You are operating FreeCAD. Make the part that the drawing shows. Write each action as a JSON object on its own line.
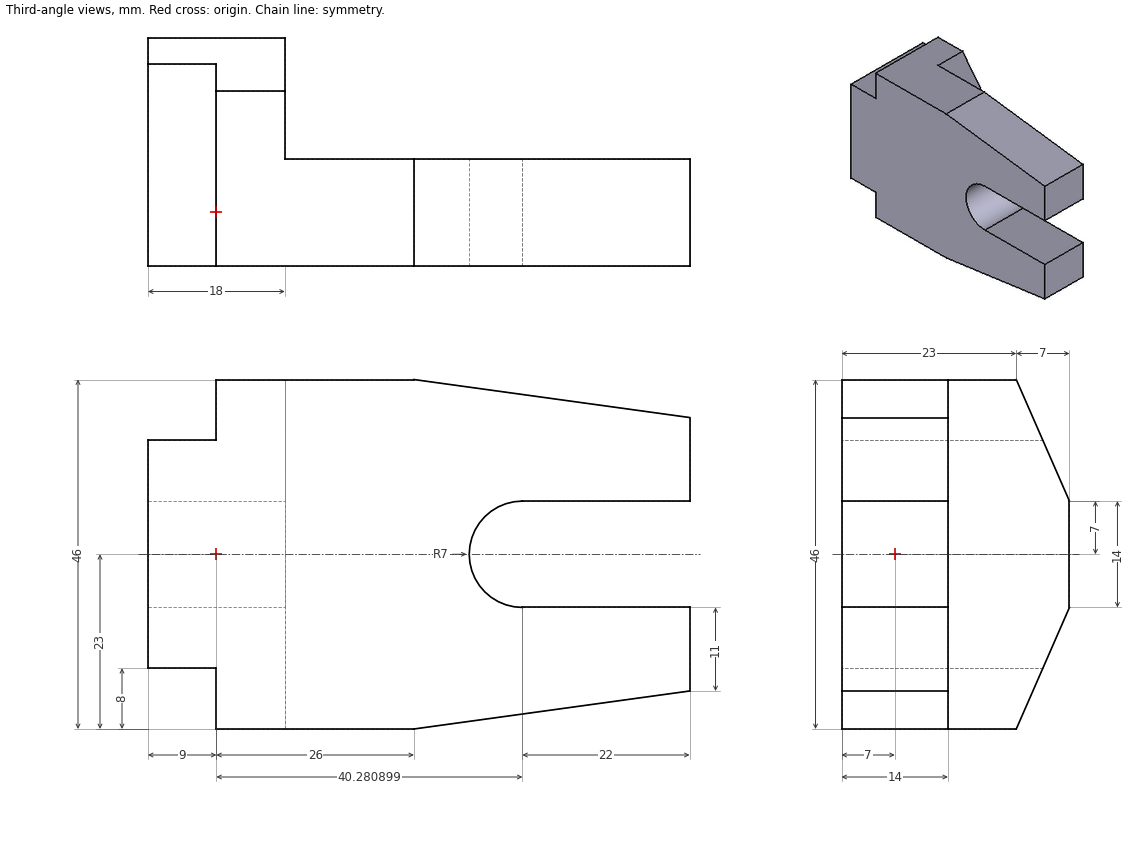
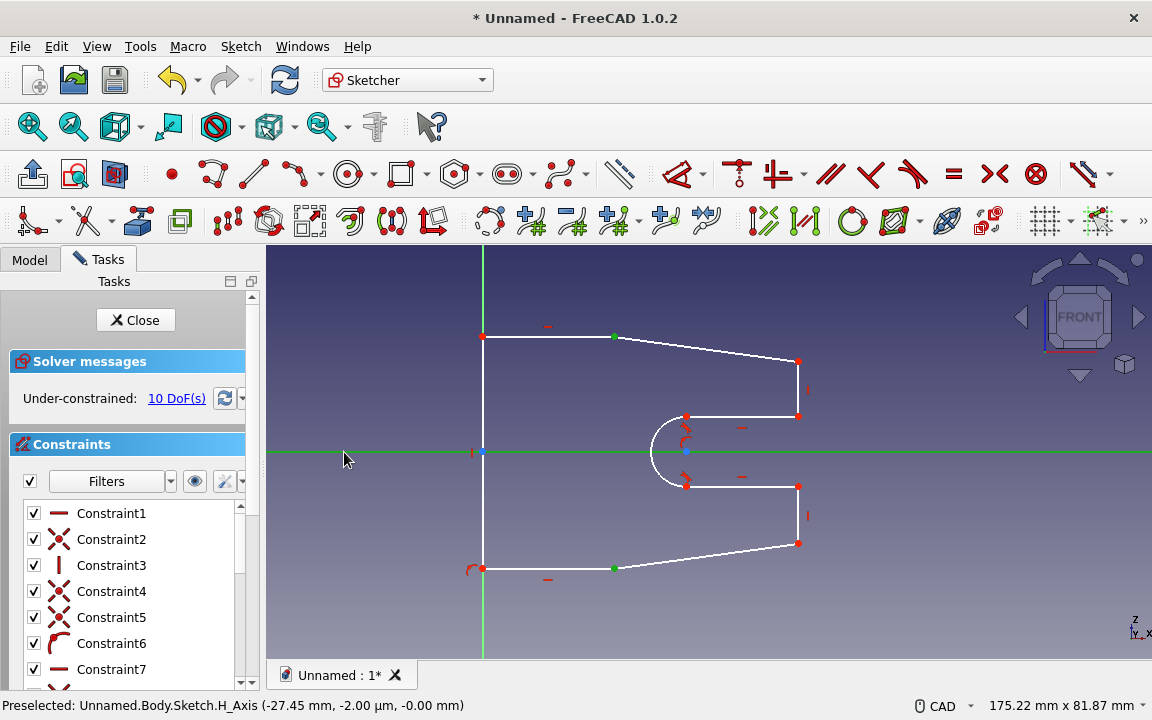
{"action": "key", "text": "s"}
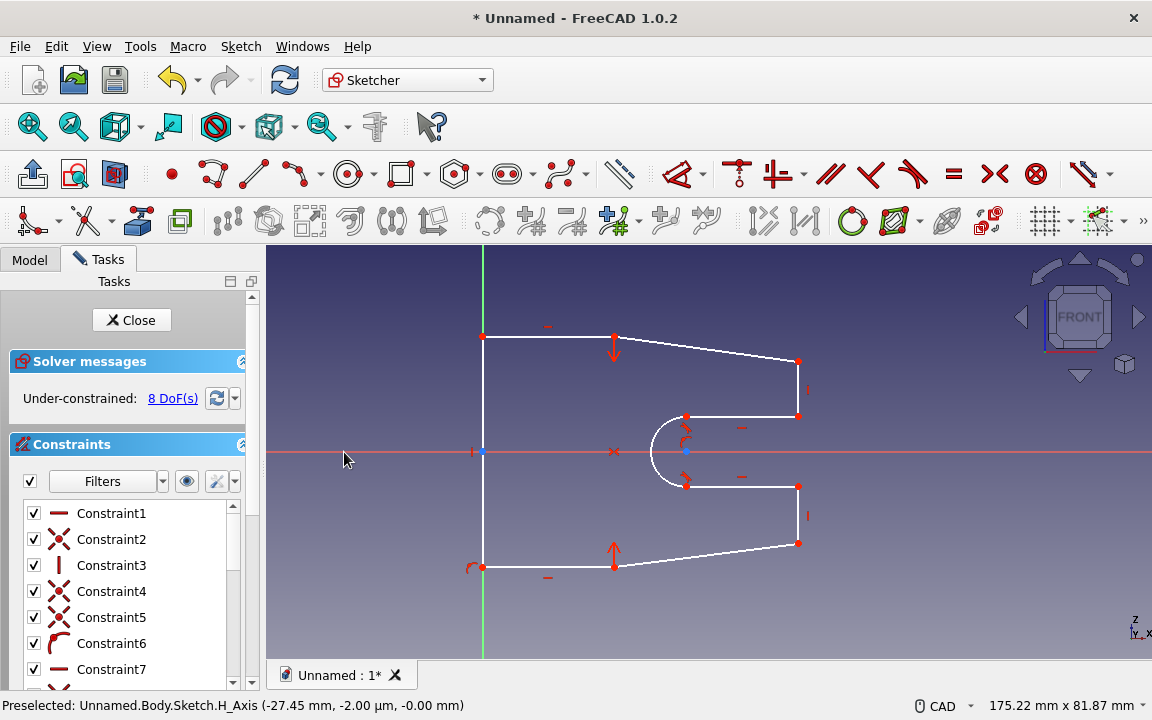
{"action": "left_click", "coordinate": [798, 544]}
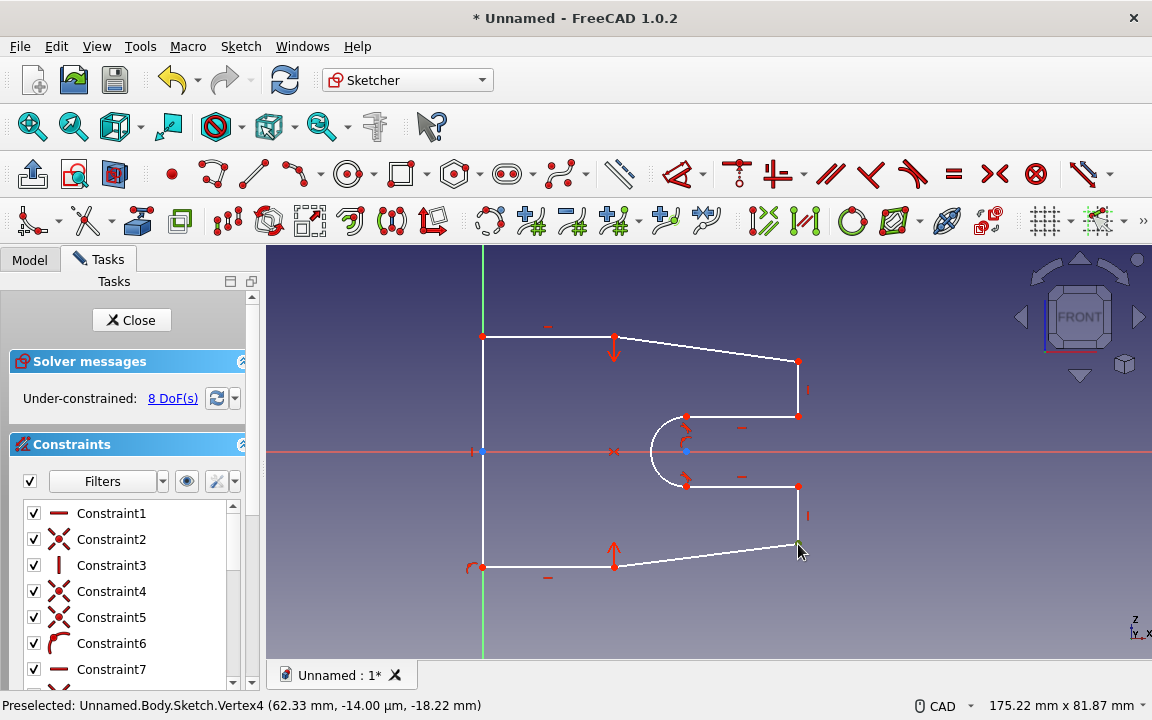
{"action": "left_click", "coordinate": [798, 362]}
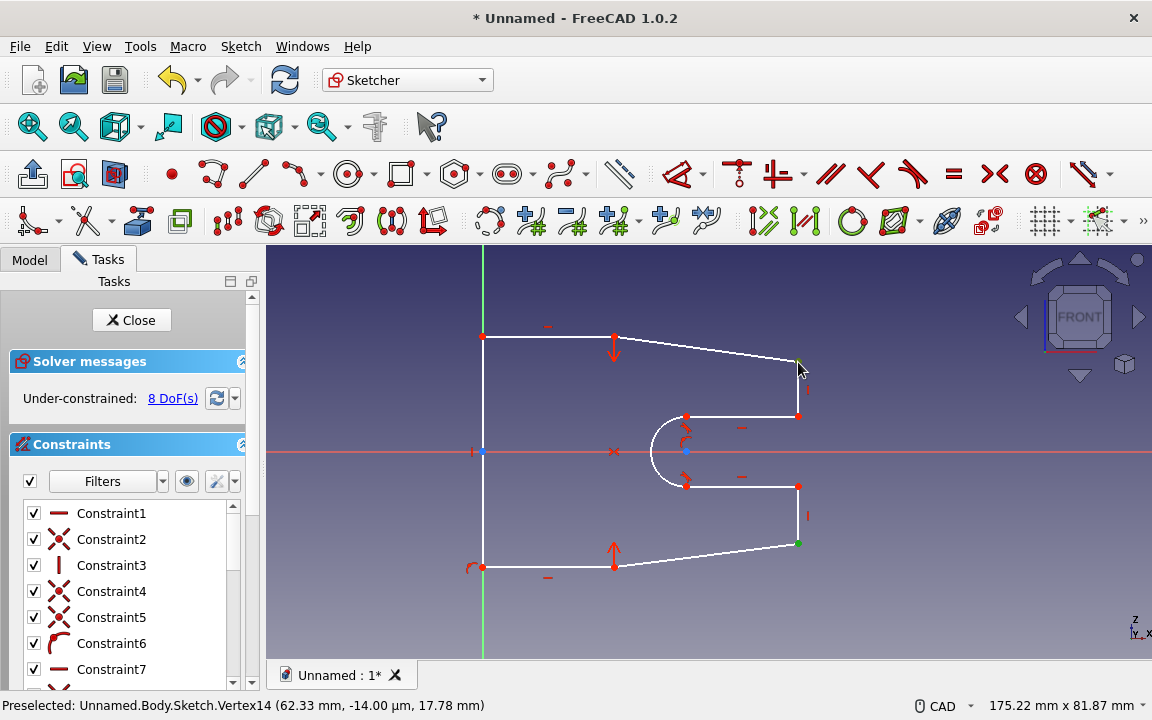
{"action": "left_click", "coordinate": [344, 452]}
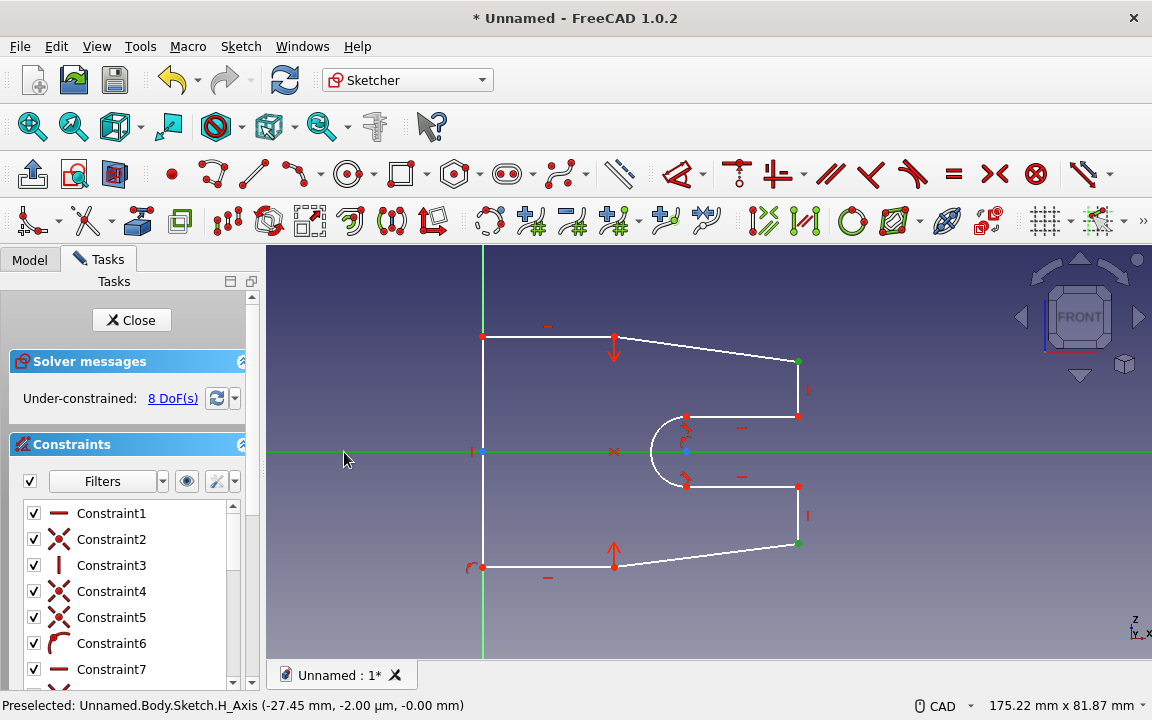
{"action": "key", "text": "s"}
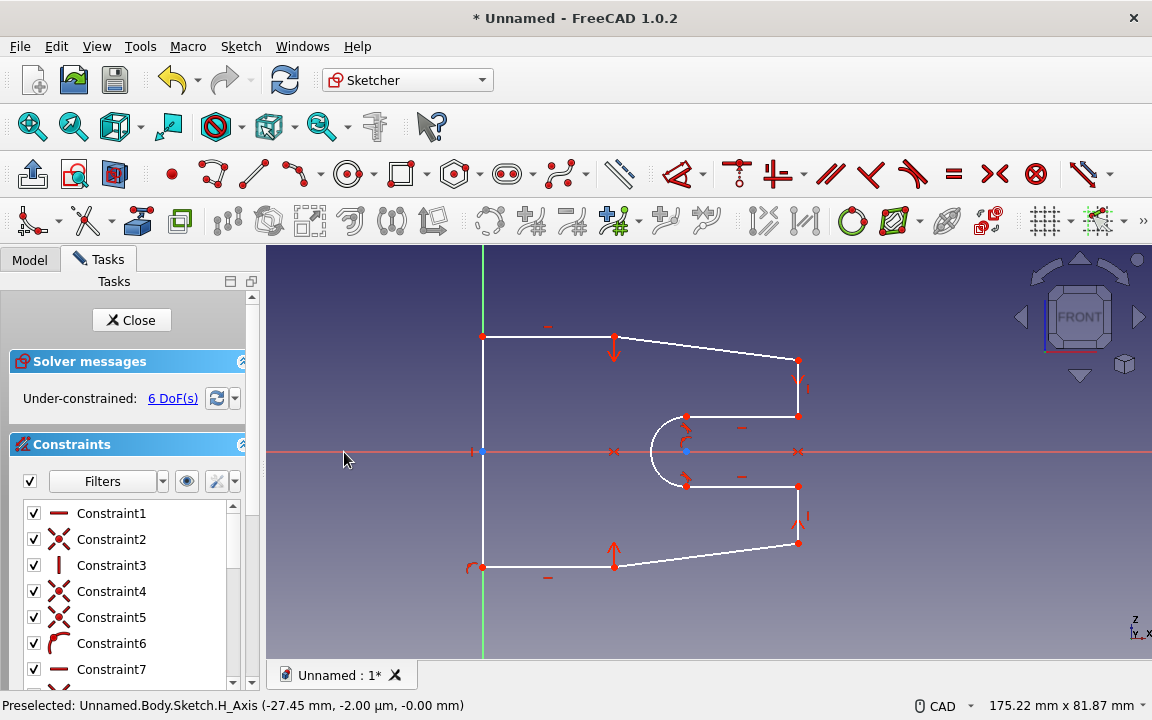
{"action": "left_click", "coordinate": [658, 431]}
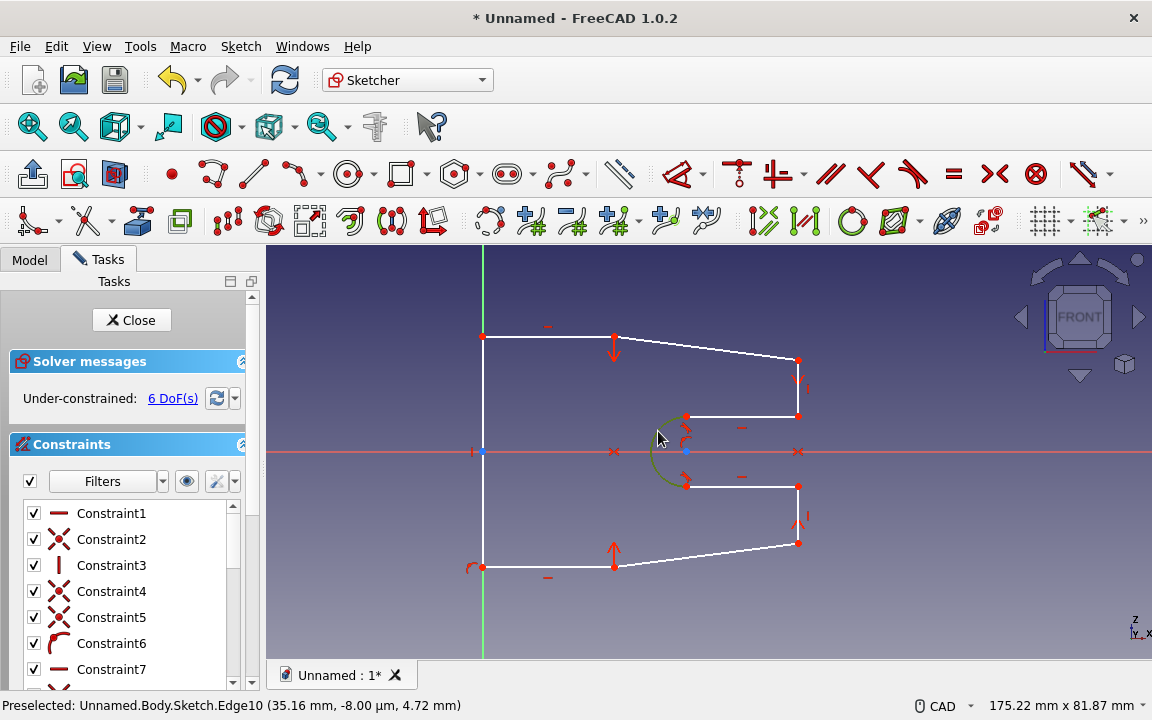
{"action": "key", "text": "k r"}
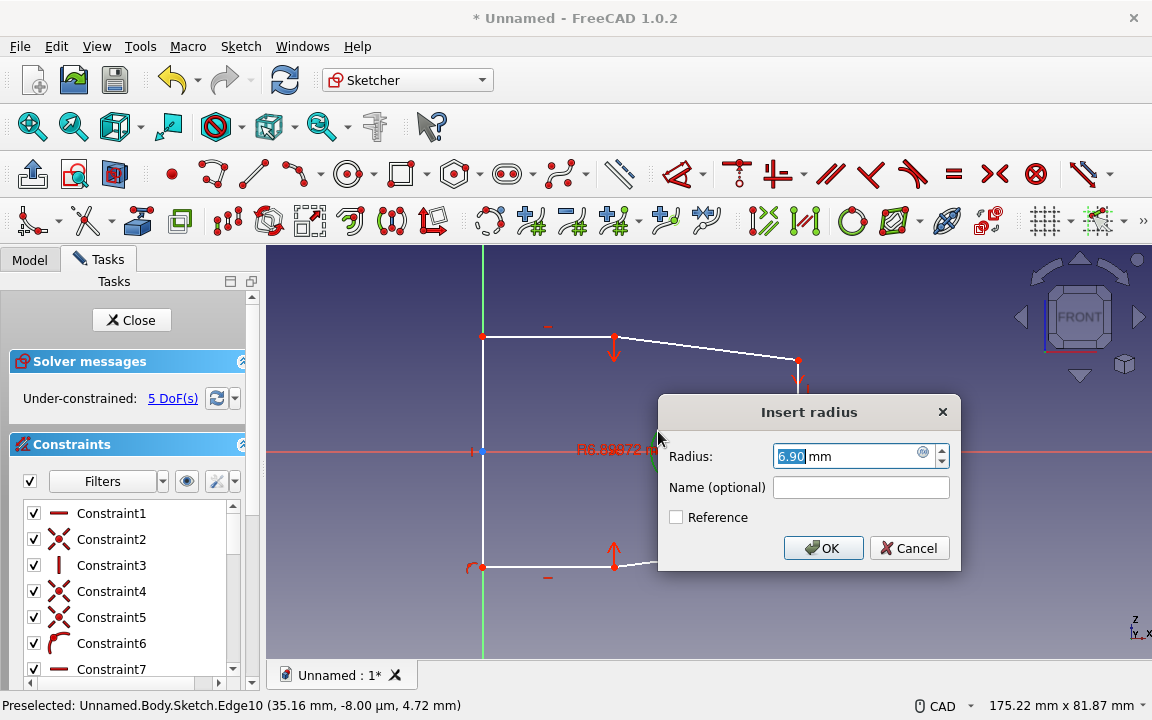
{"action": "type", "text": "7"}
{"action": "key", "text": "Return"}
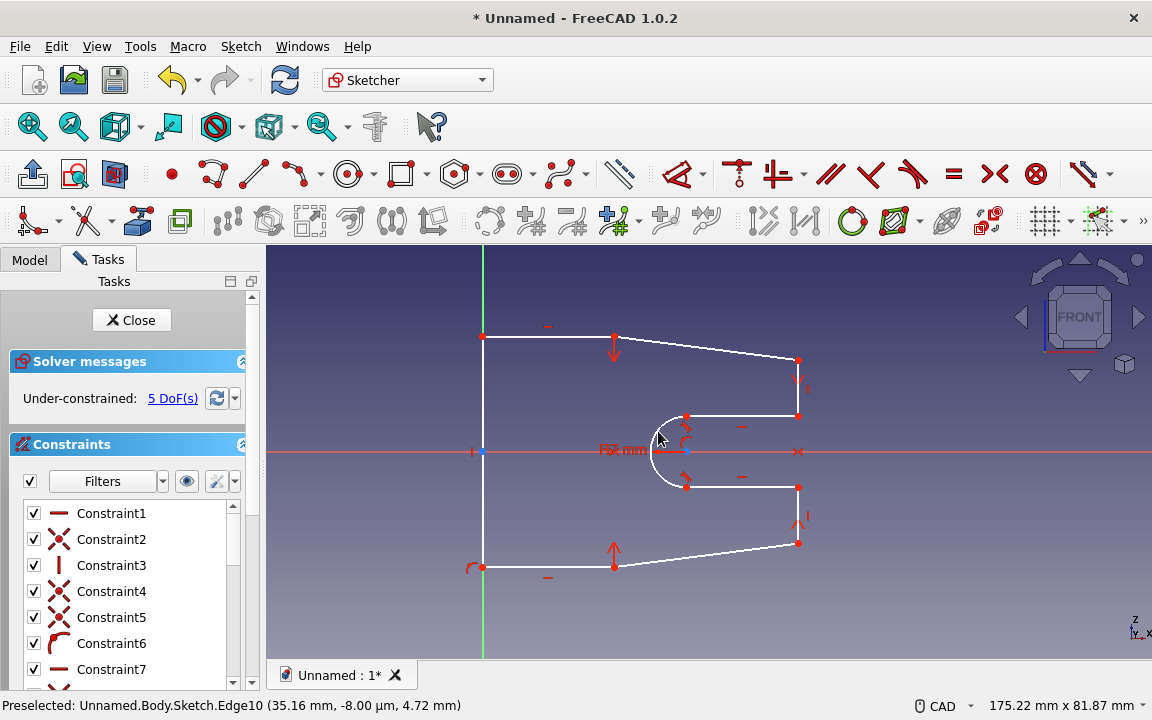
{"action": "left_click", "coordinate": [720, 487]}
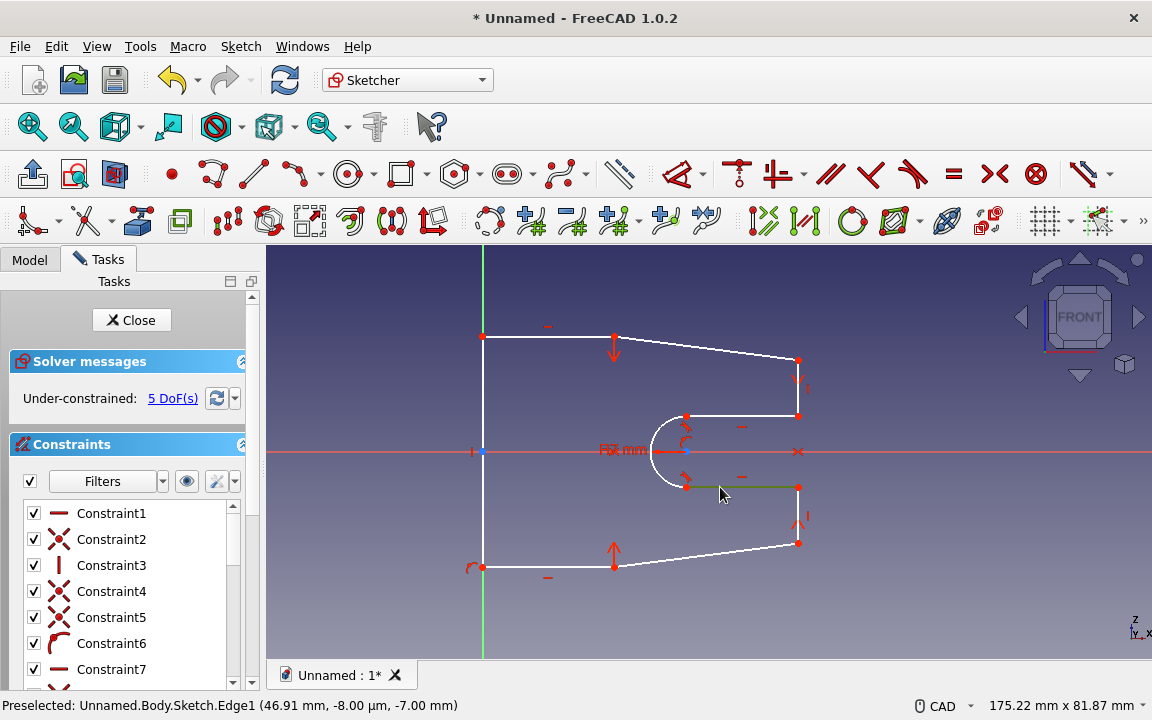
{"action": "key", "text": "l"}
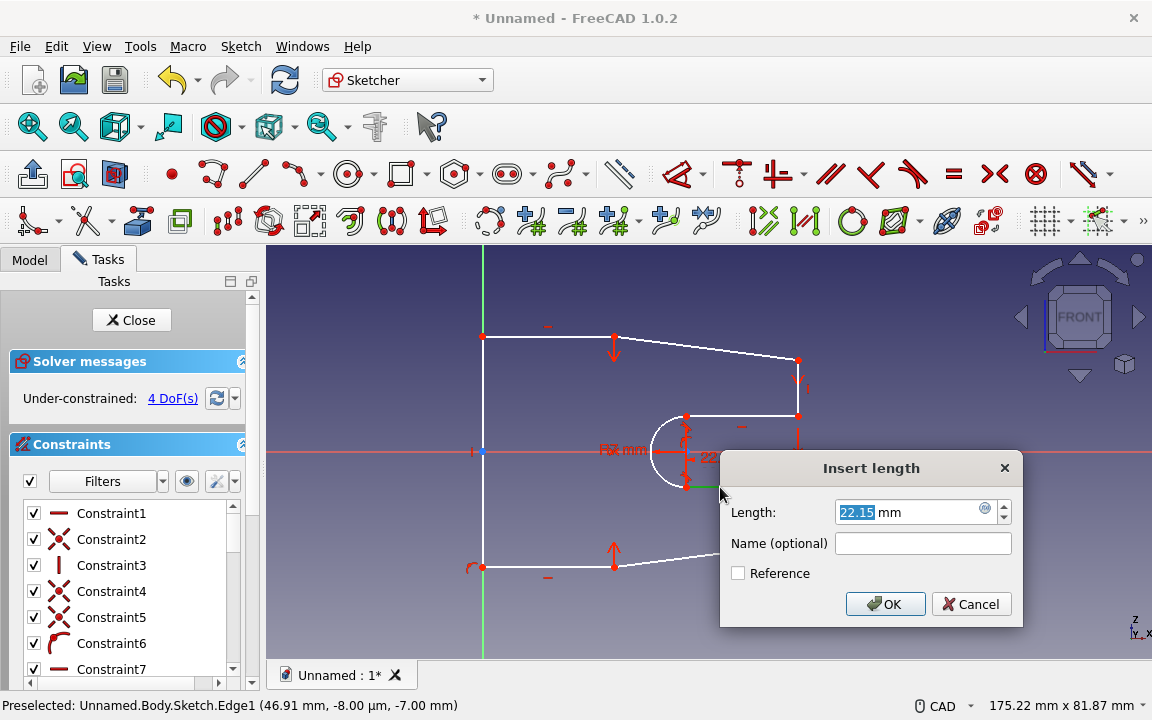
{"action": "type", "text": "22"}
{"action": "key", "text": "Return"}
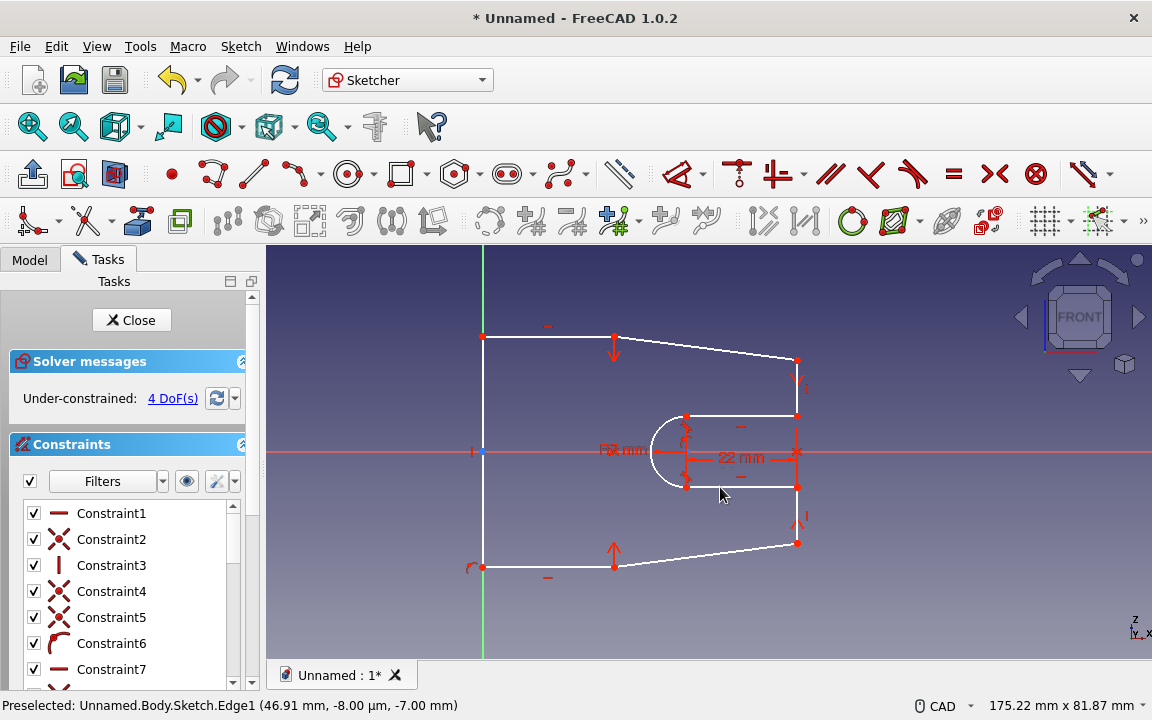
{"action": "left_click", "coordinate": [797, 504]}